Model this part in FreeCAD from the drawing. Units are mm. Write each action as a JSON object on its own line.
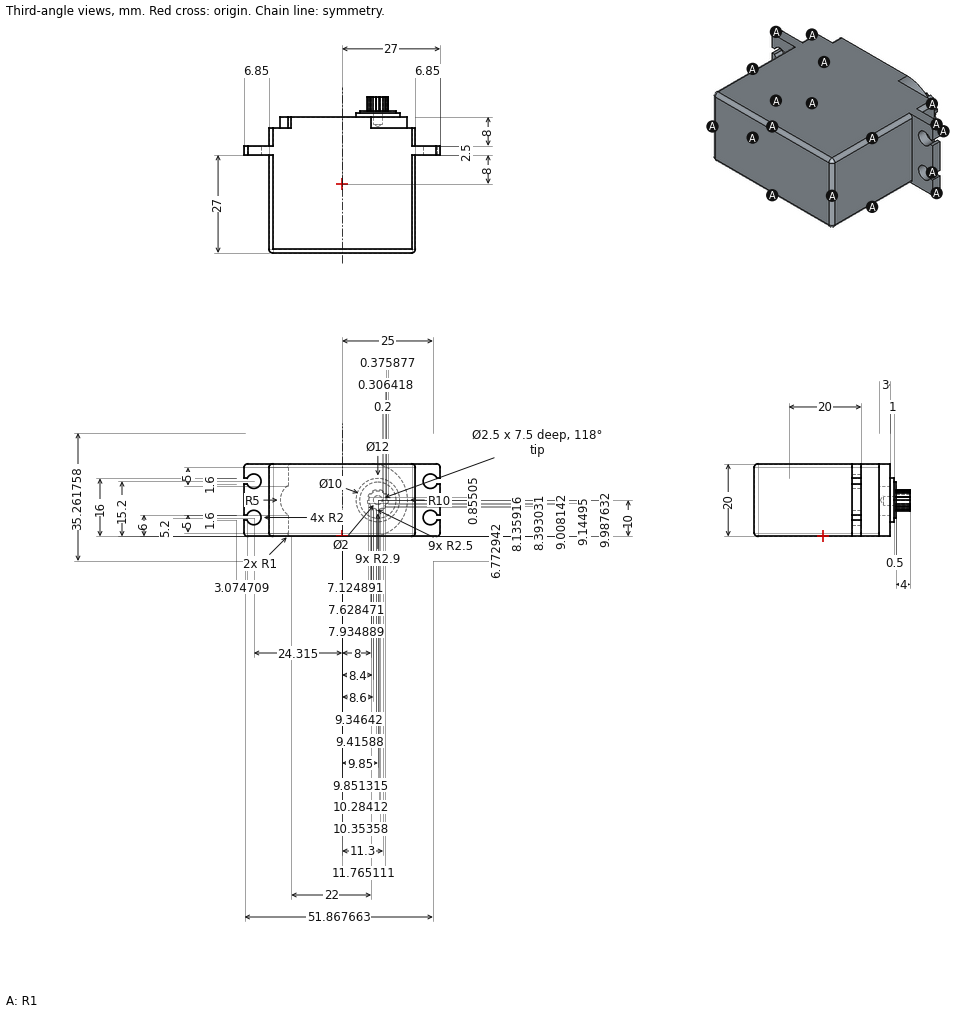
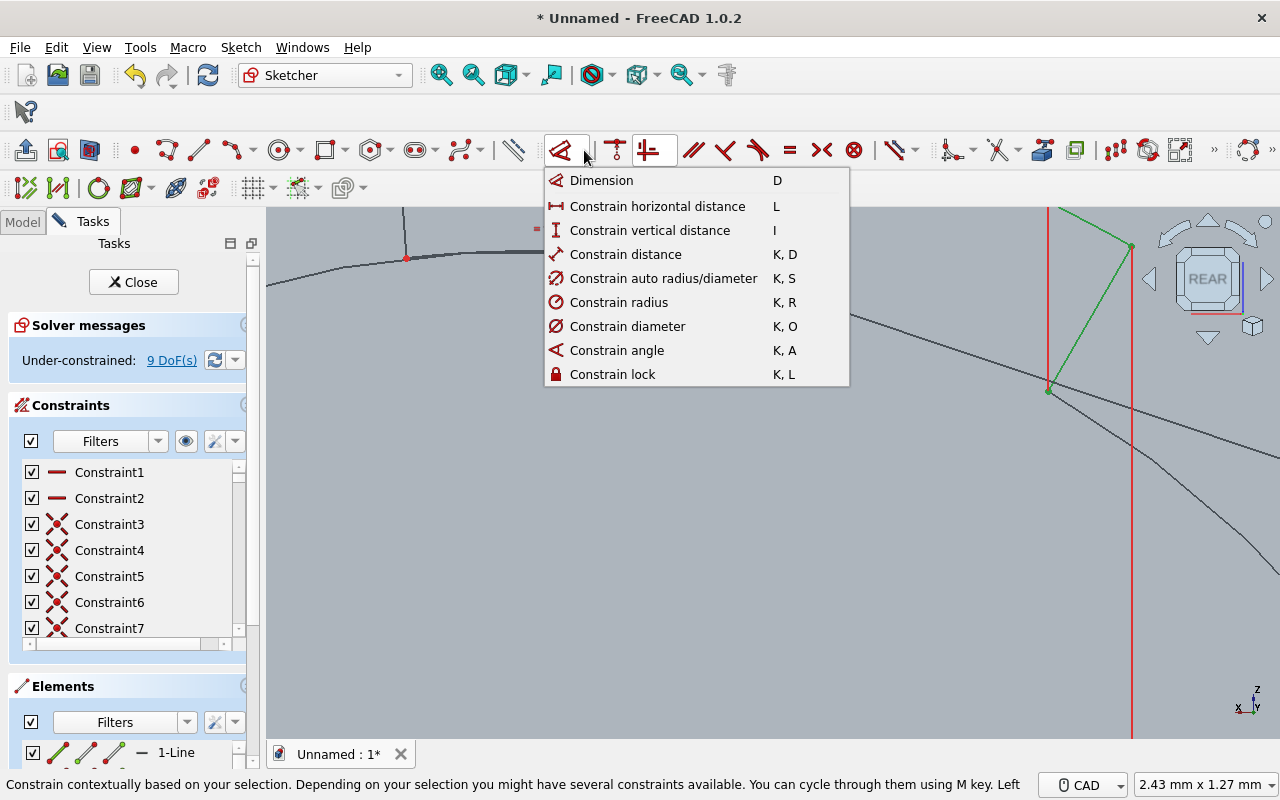
{"action": "left_click", "coordinate": [697, 206]}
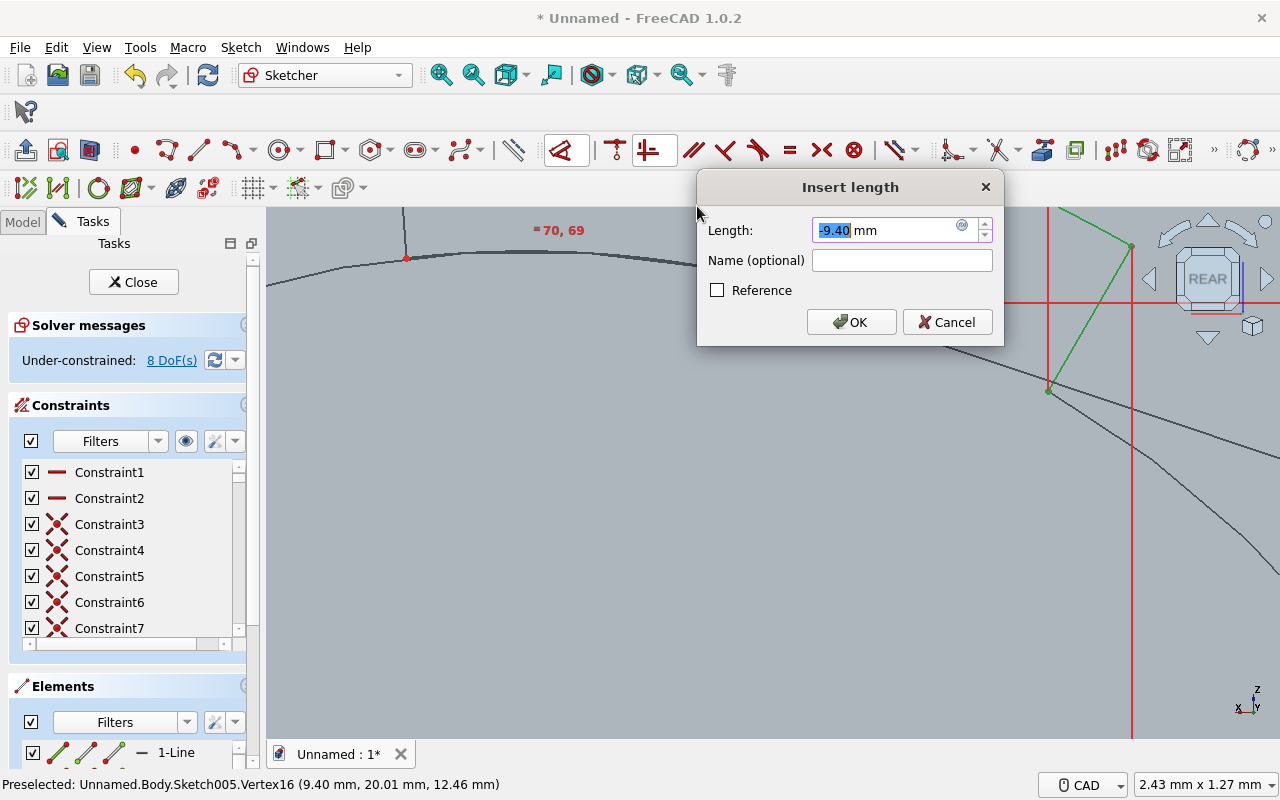
{"action": "type", "text": "-7.934889"}
{"action": "key", "text": "Return"}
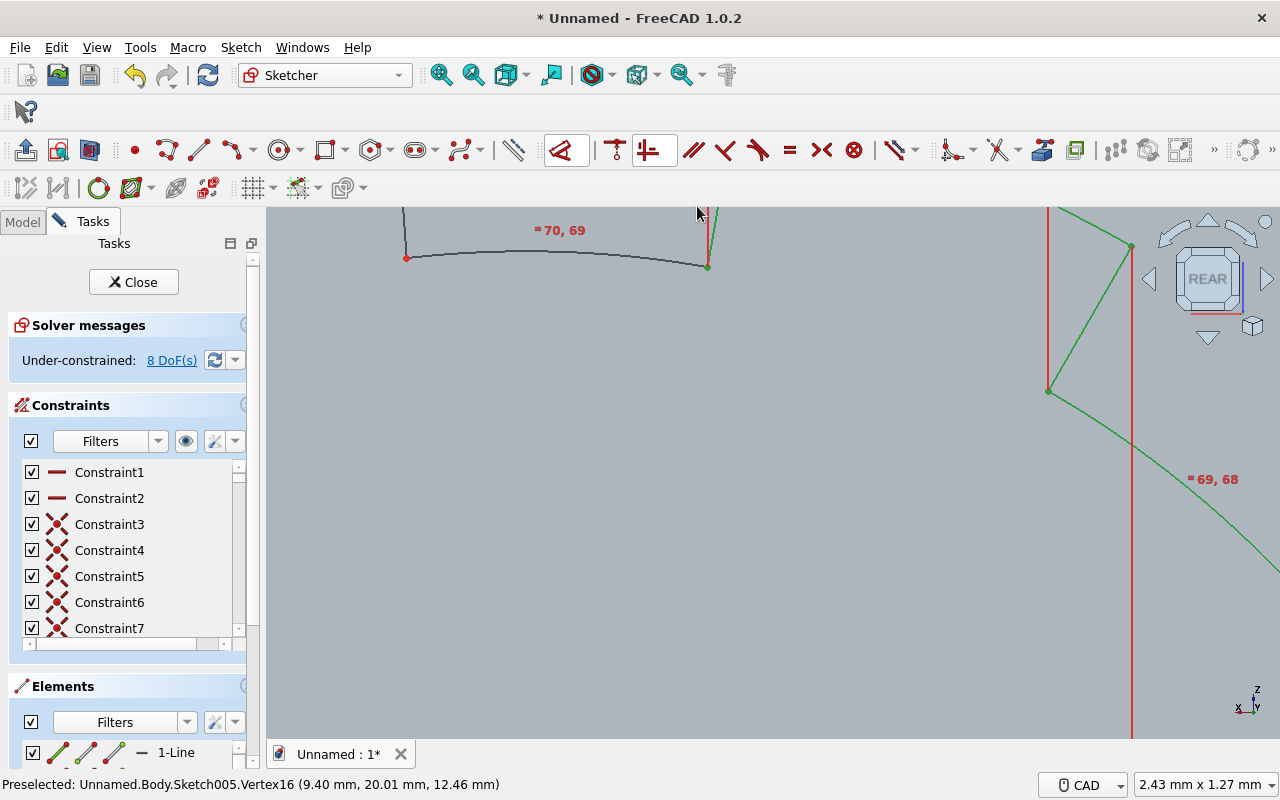
{"action": "scroll", "coordinate": [622, 323], "scroll_direction": "down", "scroll_amount": 14}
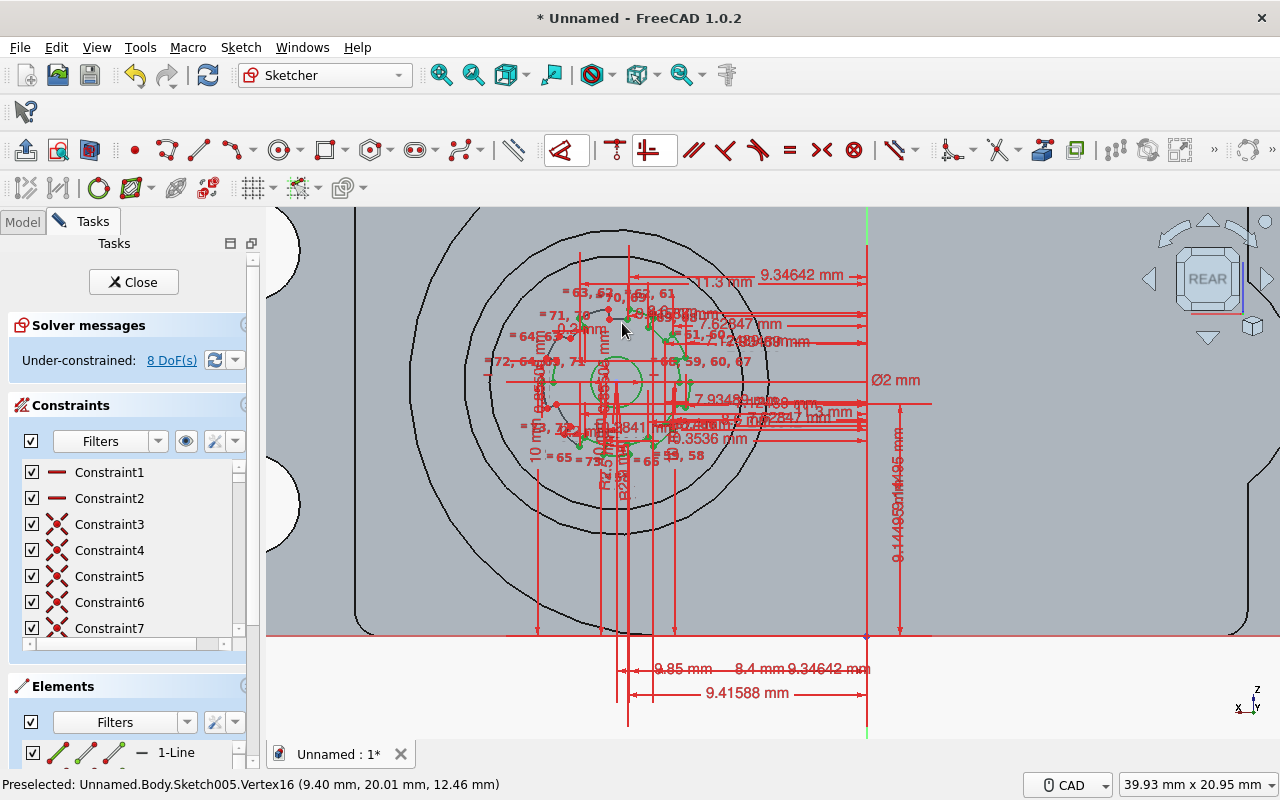
{"action": "left_click", "coordinate": [609, 319]}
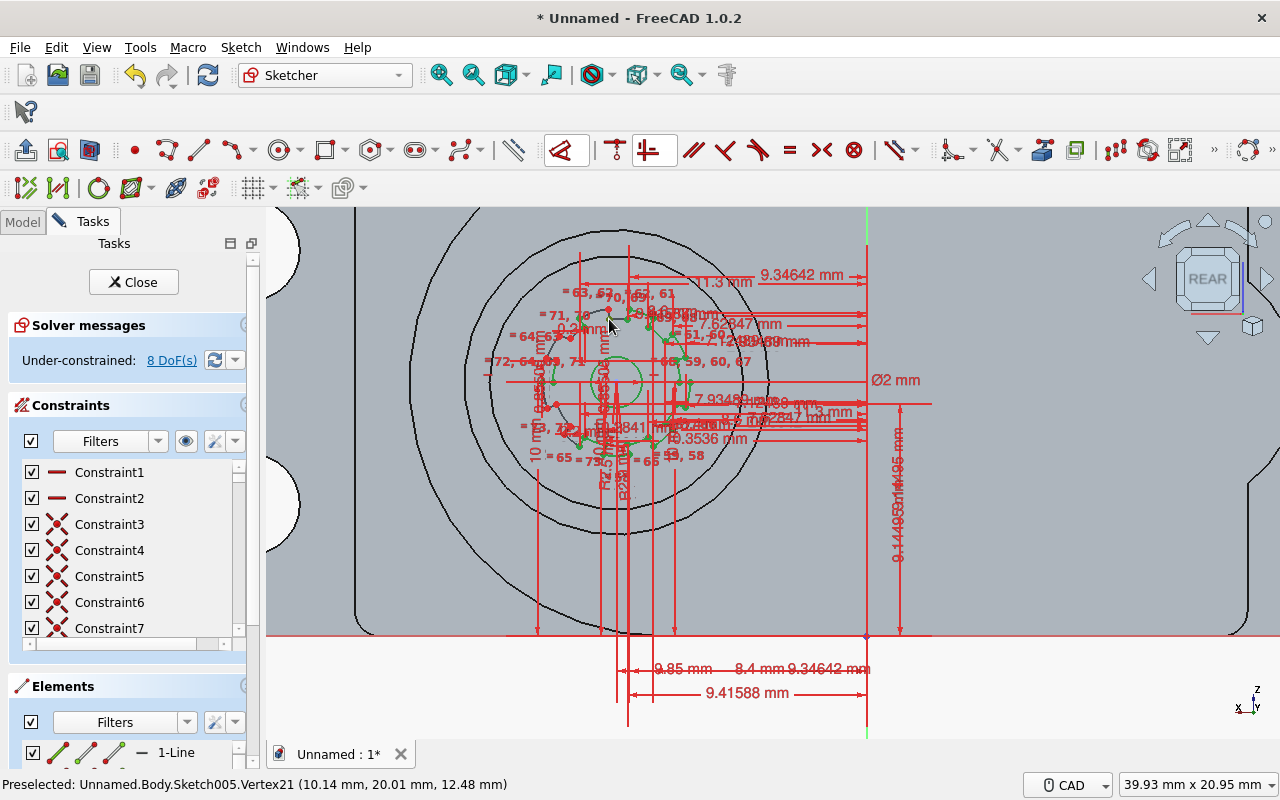
{"action": "key", "text": "l"}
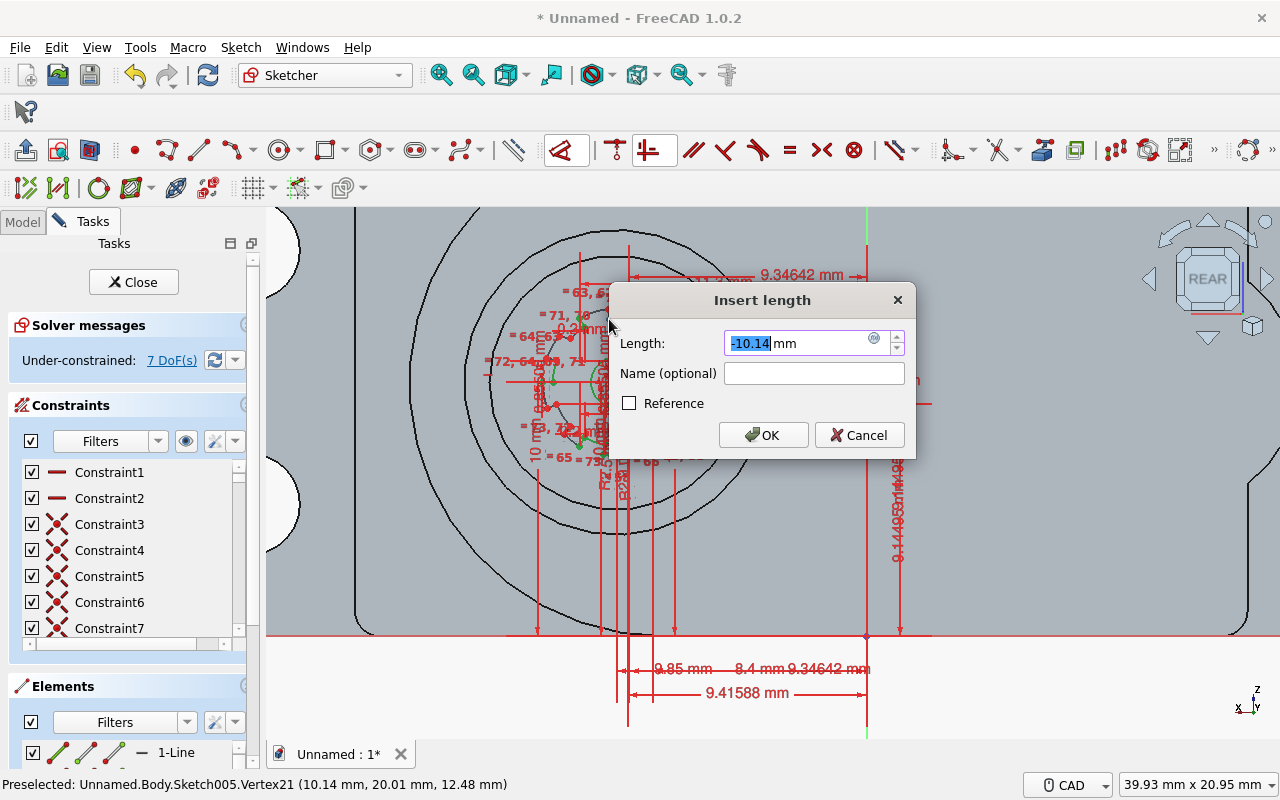
{"action": "type", "text": "-10.28412"}
{"action": "key", "text": "Return"}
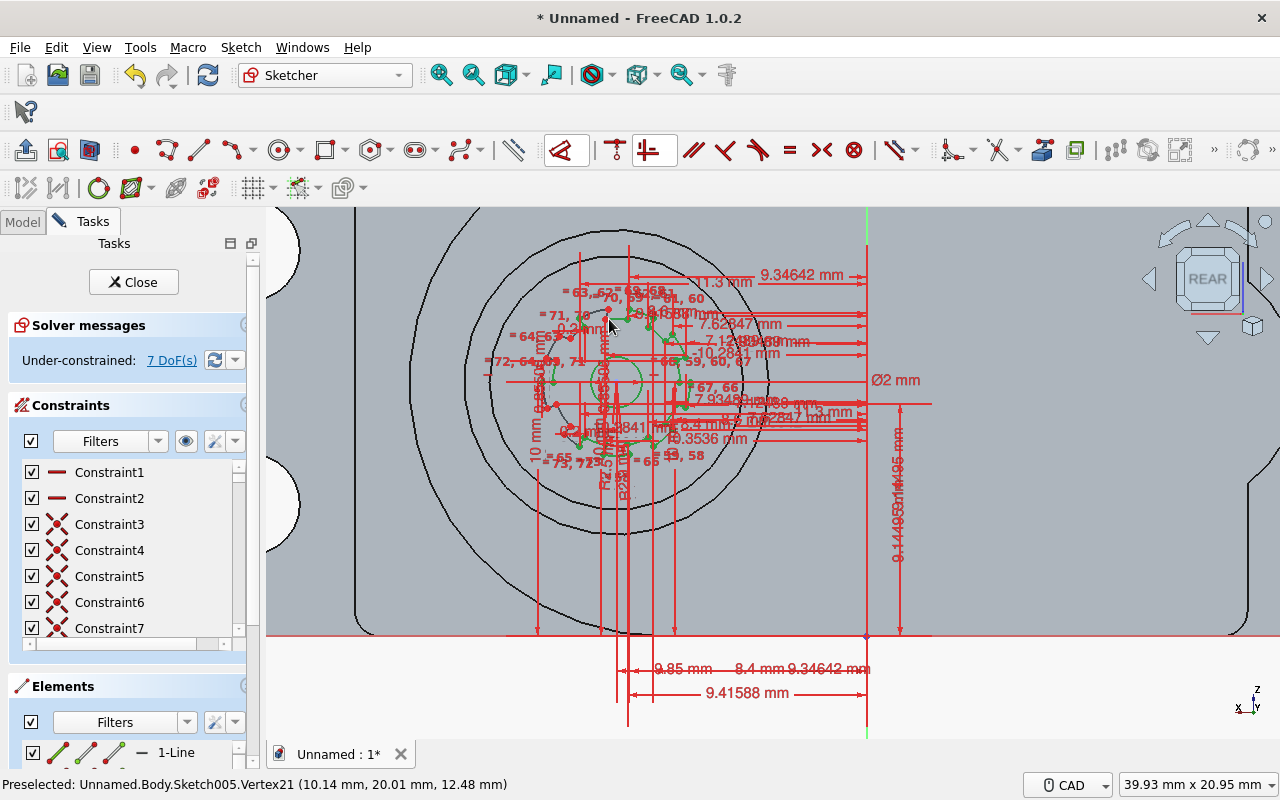
{"action": "left_click", "coordinate": [609, 309]}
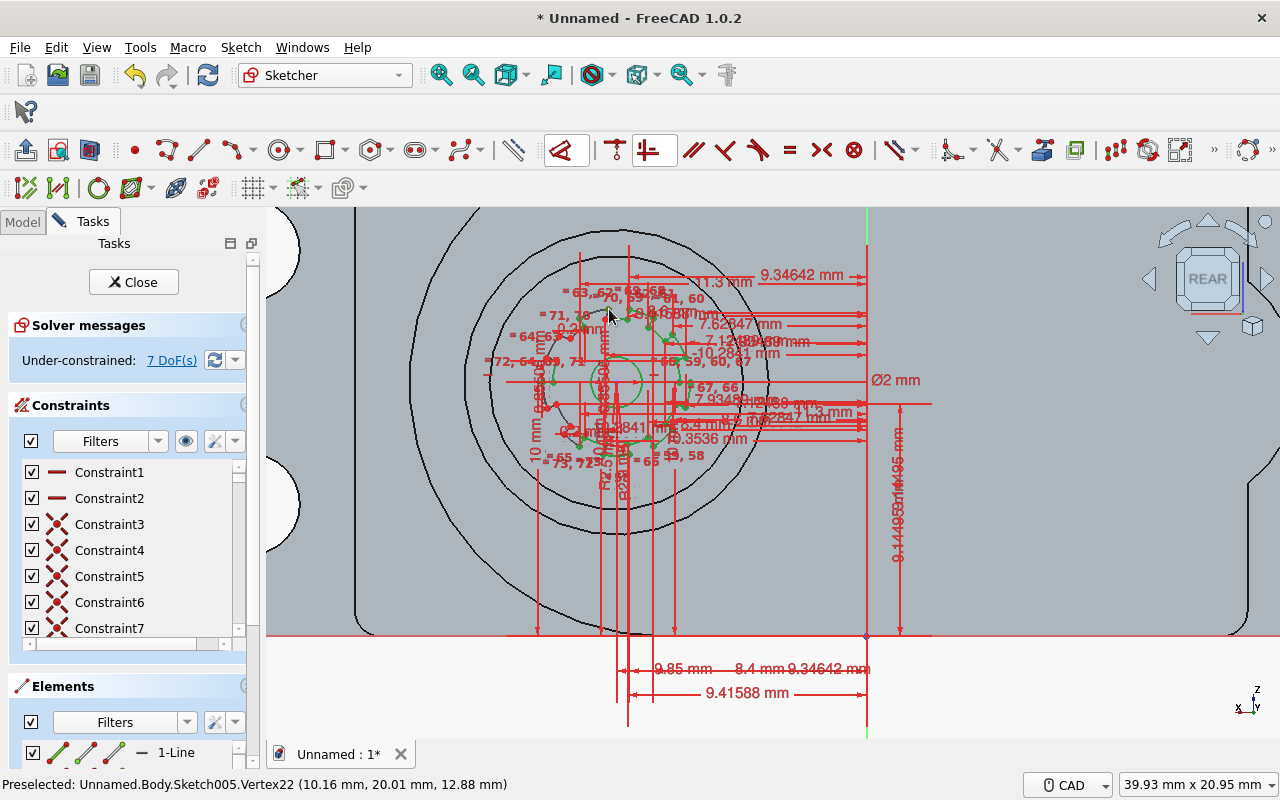
{"action": "left_click", "coordinate": [584, 150]}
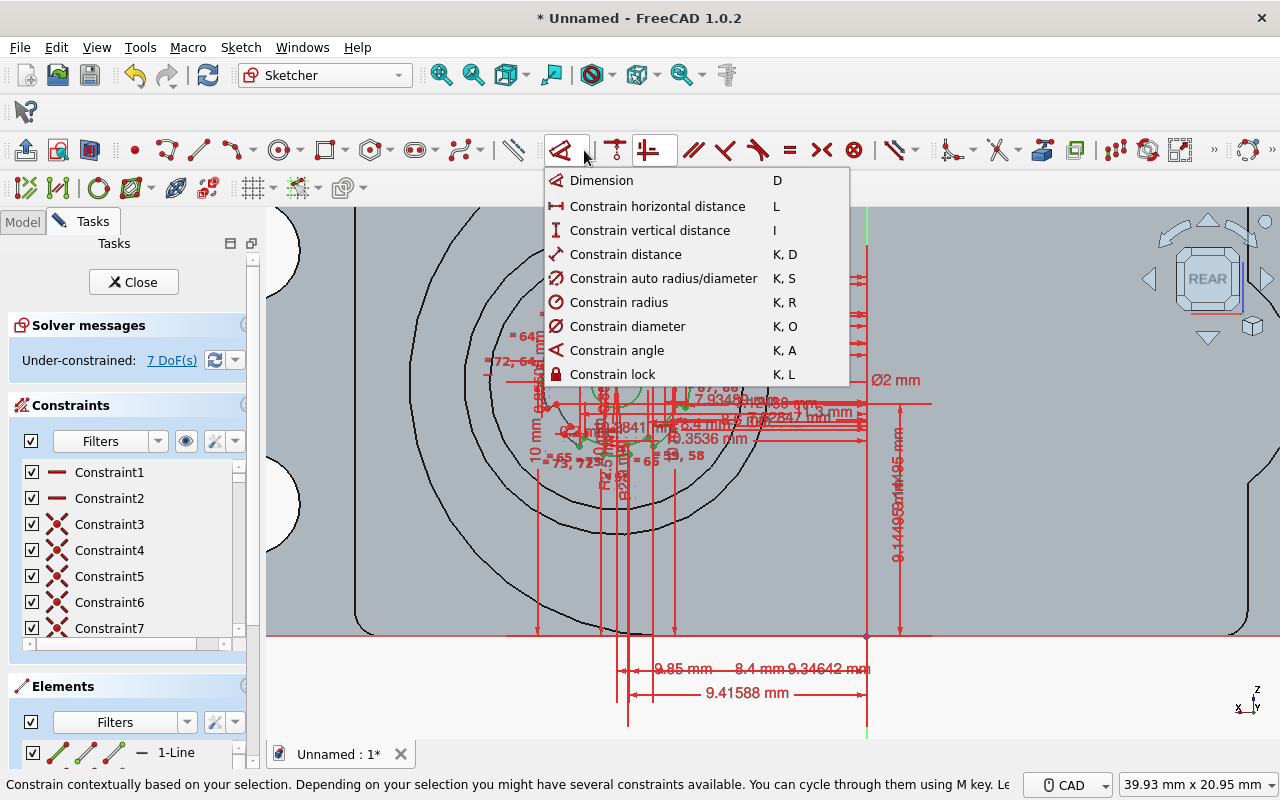
{"action": "left_click", "coordinate": [697, 206]}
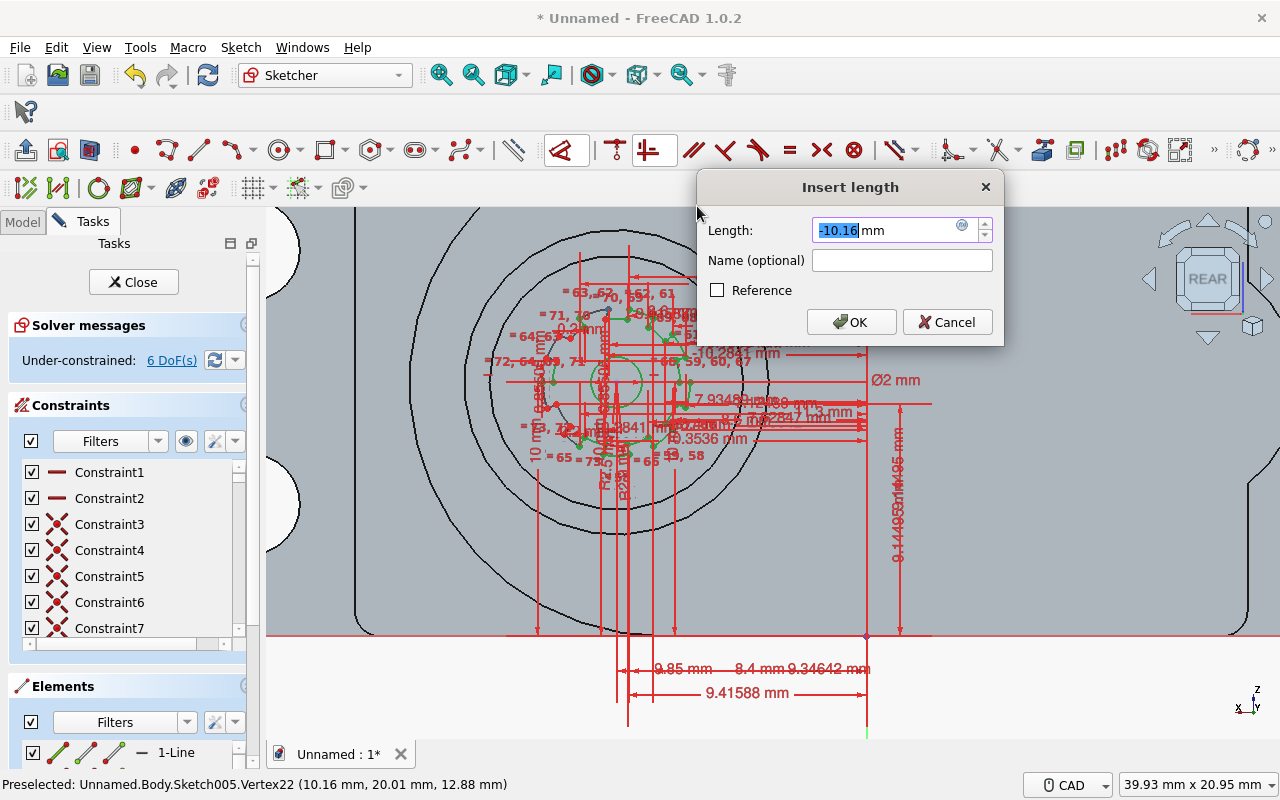
{"action": "type", "text": "-10.35358"}
{"action": "key", "text": "Return"}